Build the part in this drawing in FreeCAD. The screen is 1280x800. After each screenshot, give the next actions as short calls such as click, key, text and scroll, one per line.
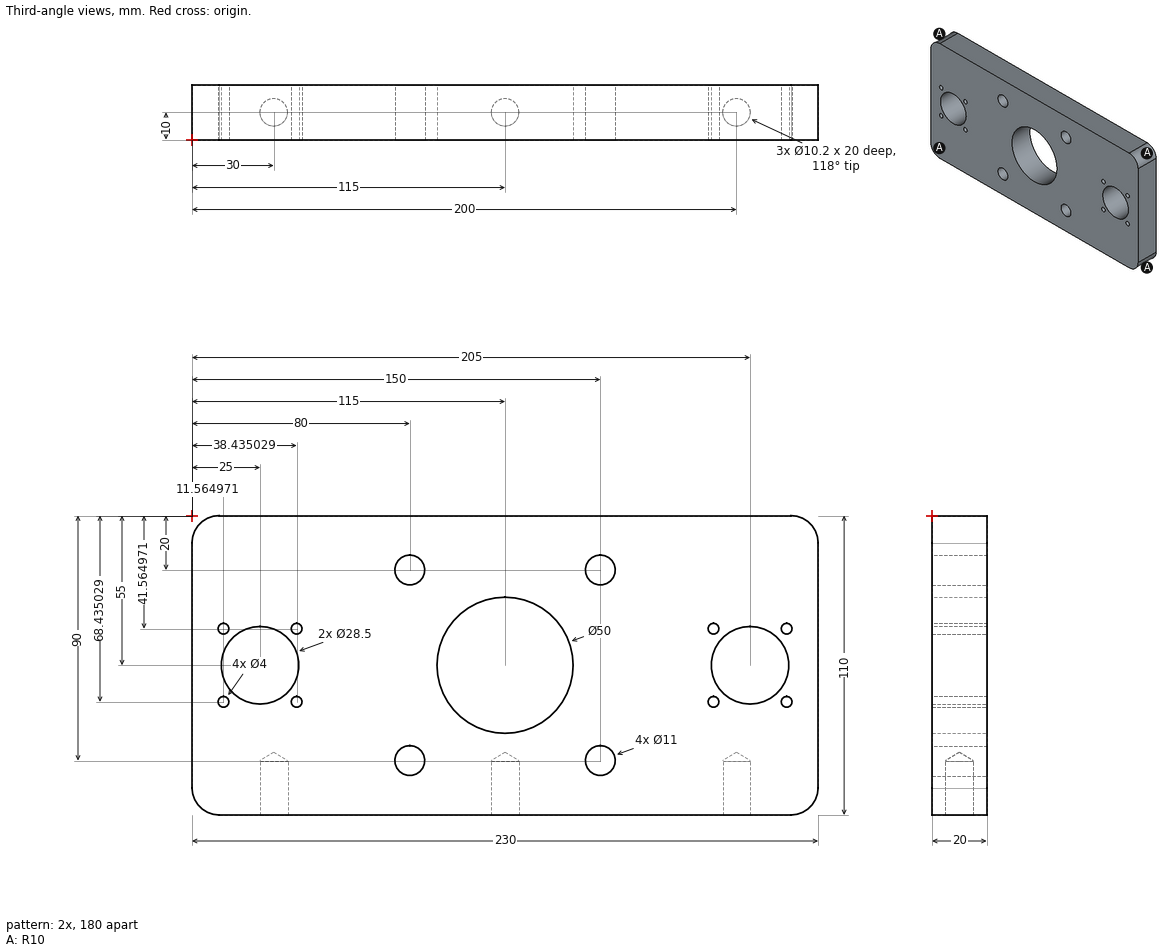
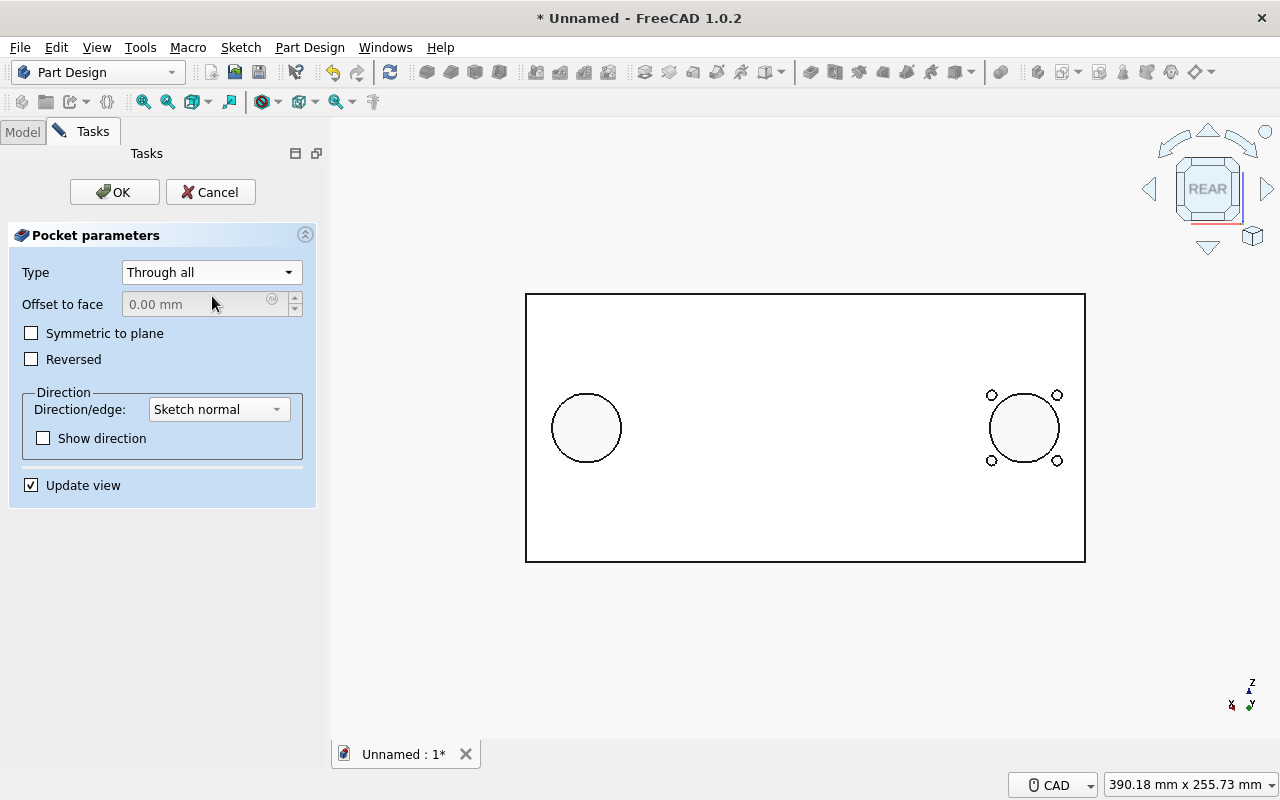
click(115, 192)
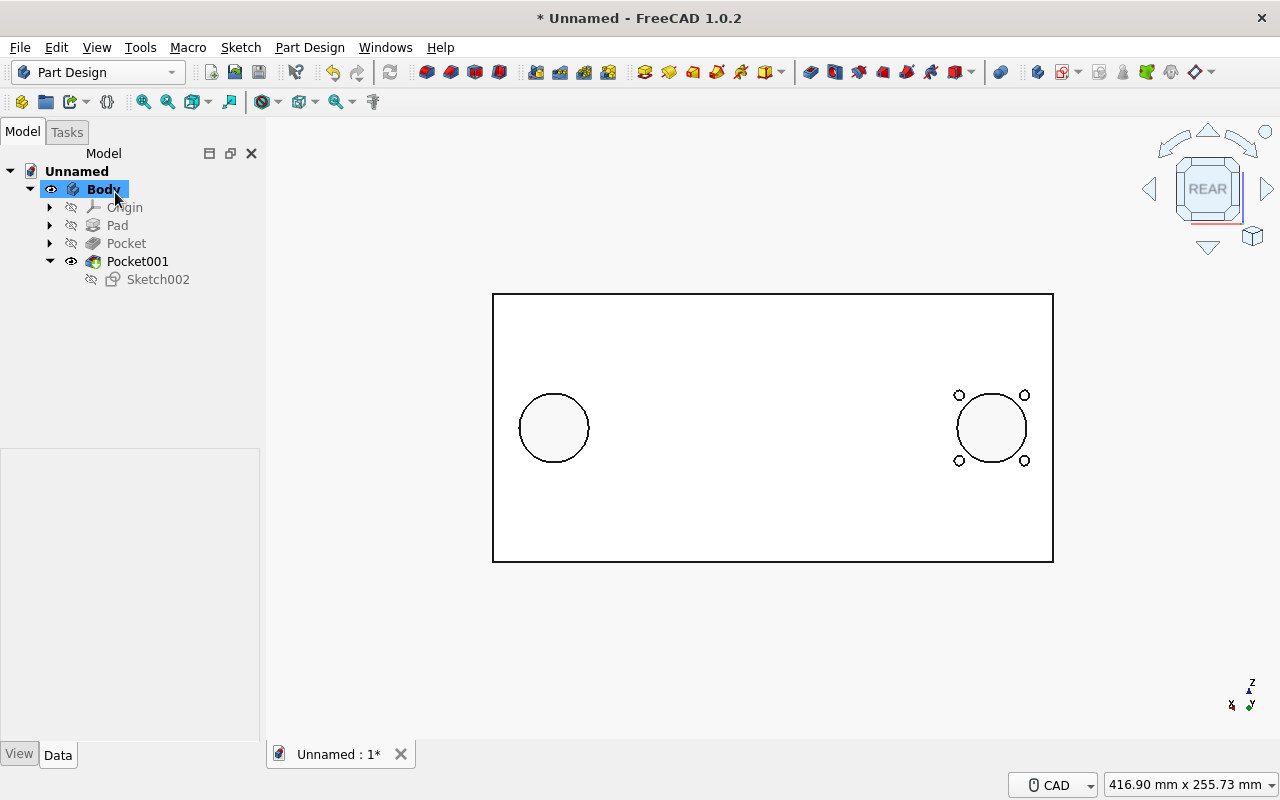
click(116, 261)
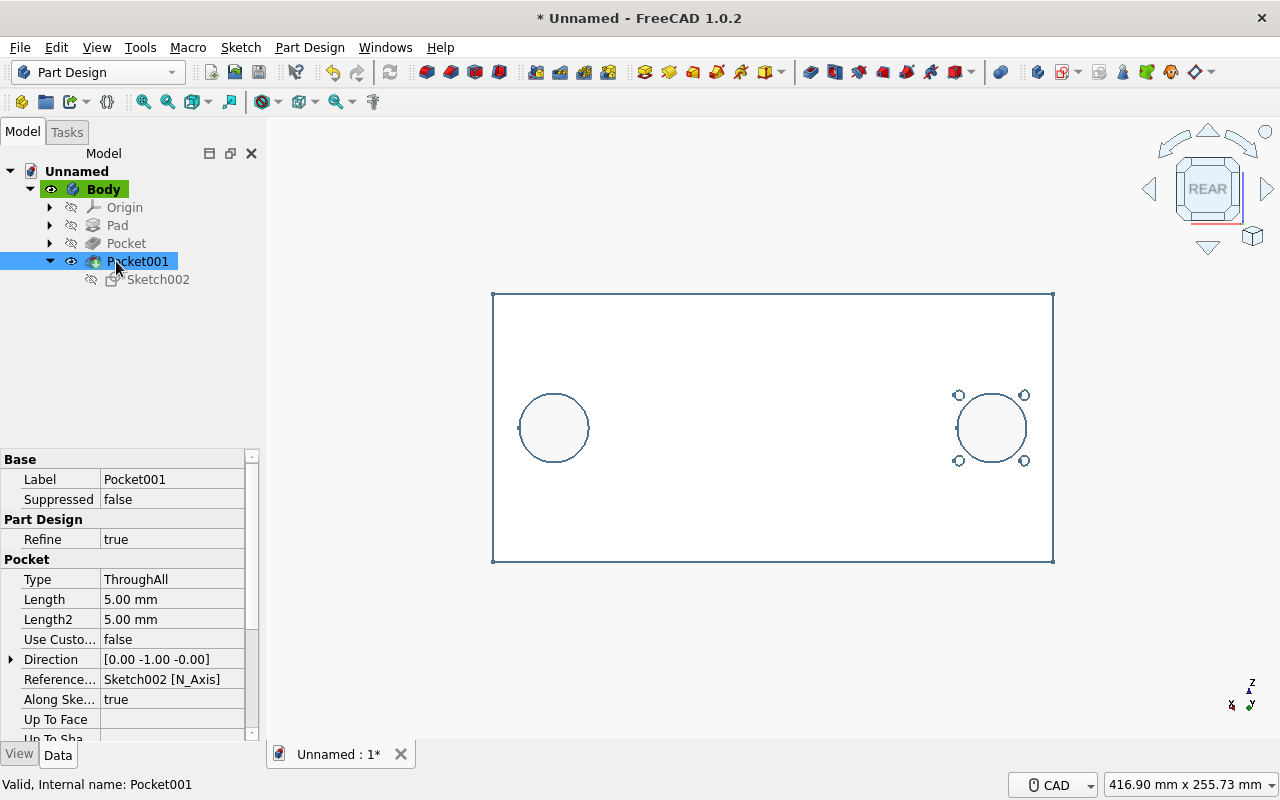
click(560, 72)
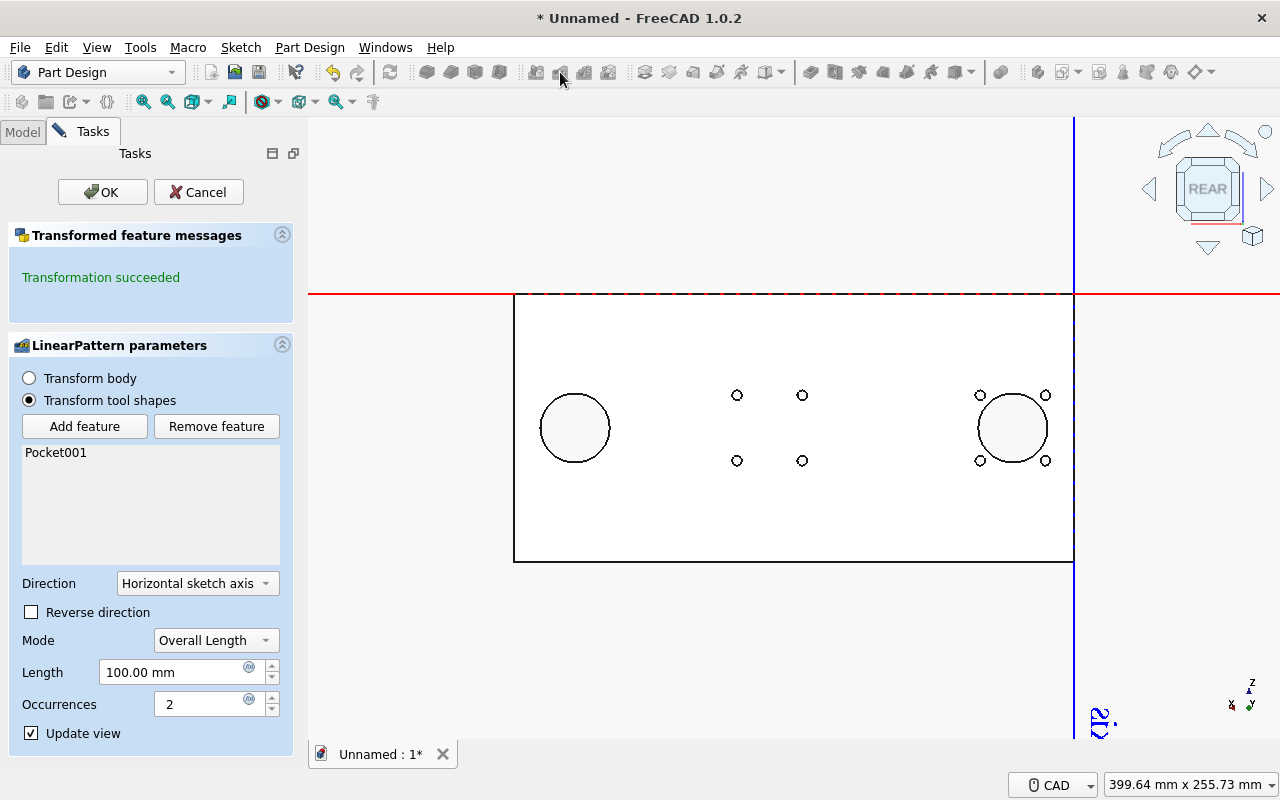
click(198, 584)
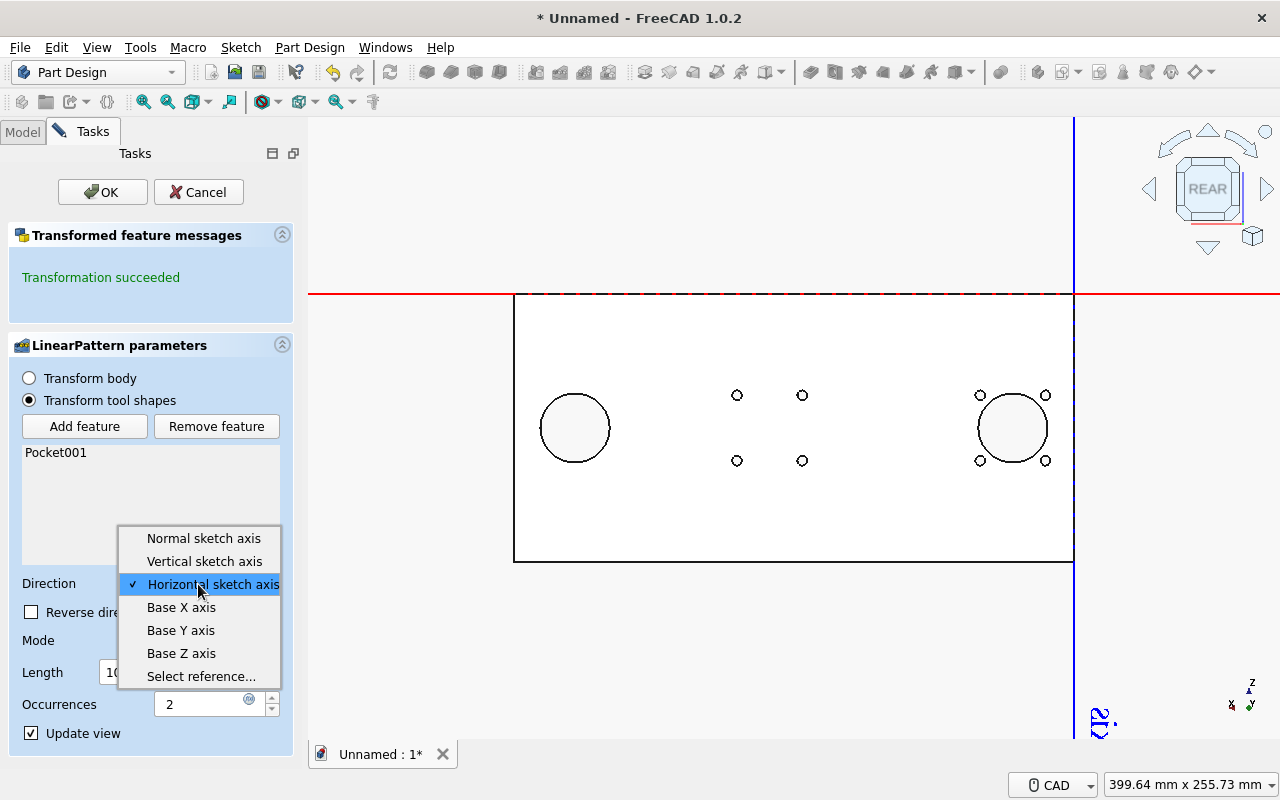
click(198, 608)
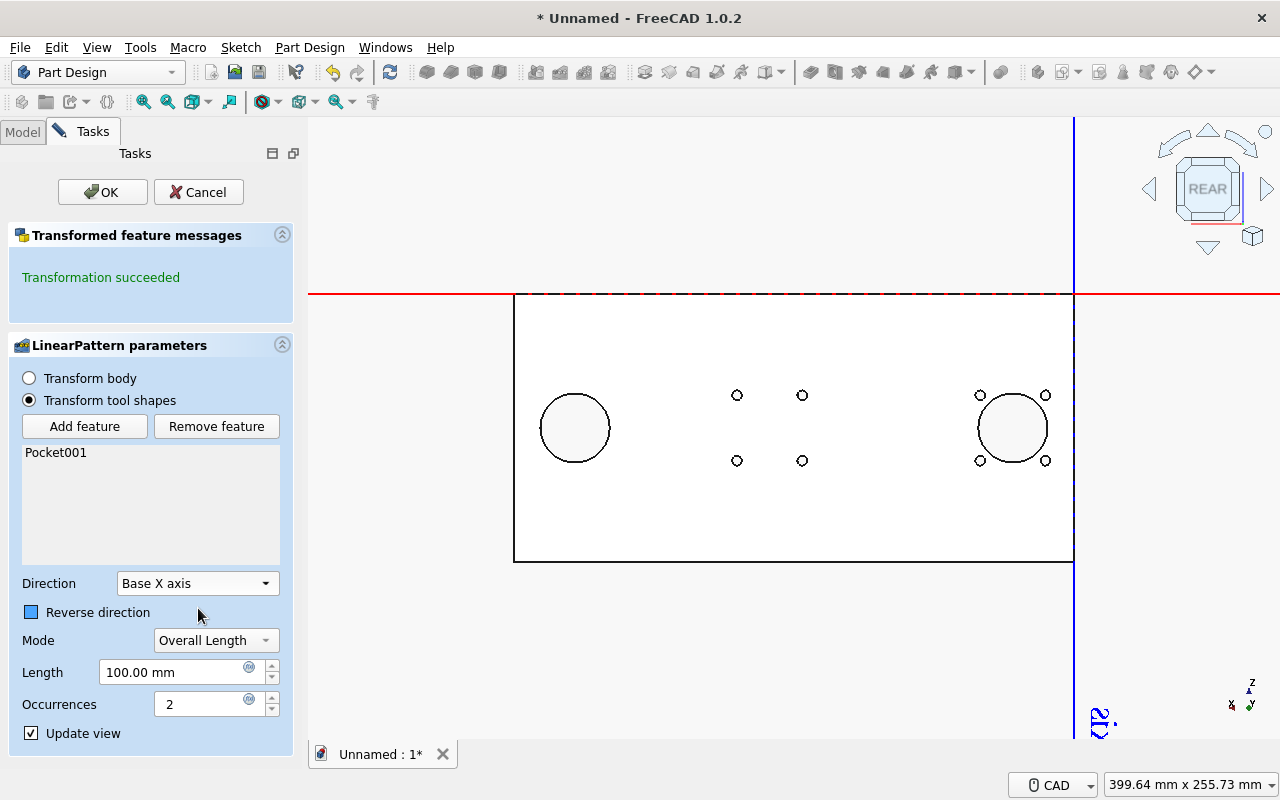
click(217, 640)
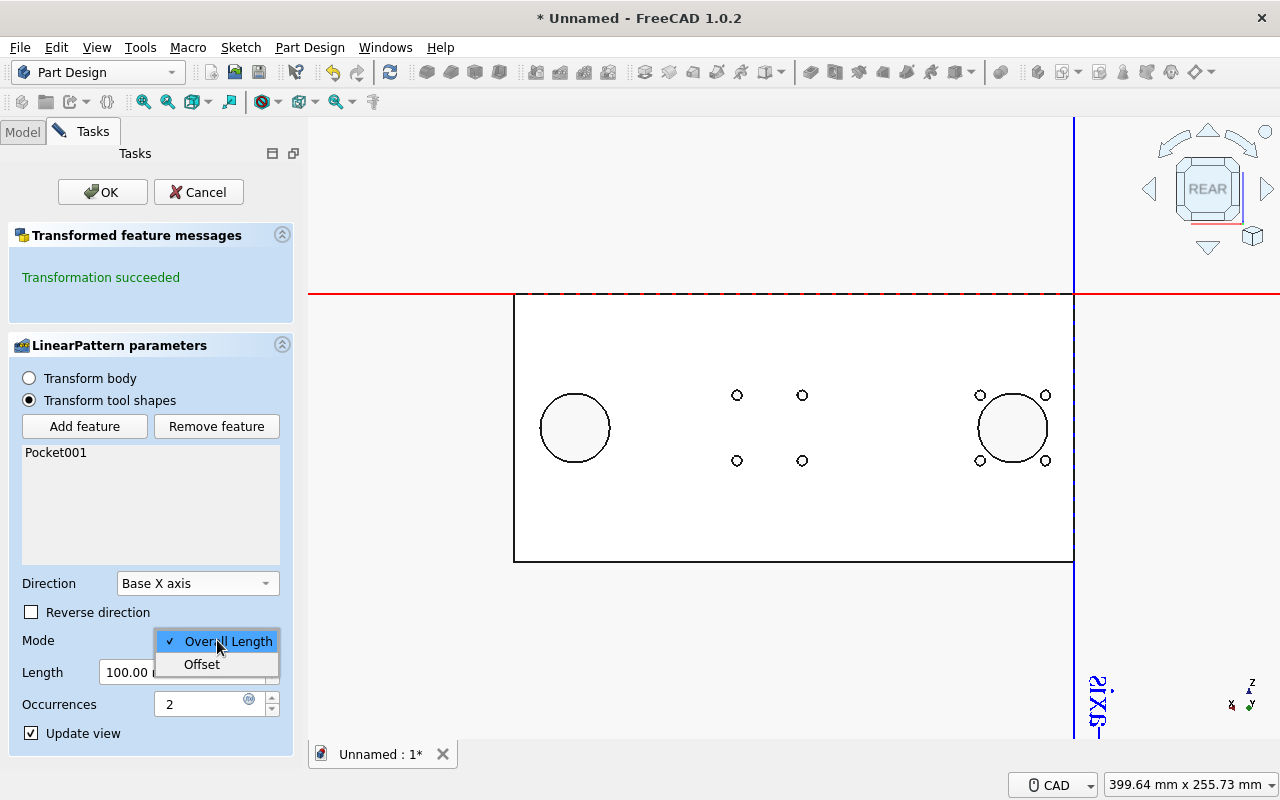
click(216, 664)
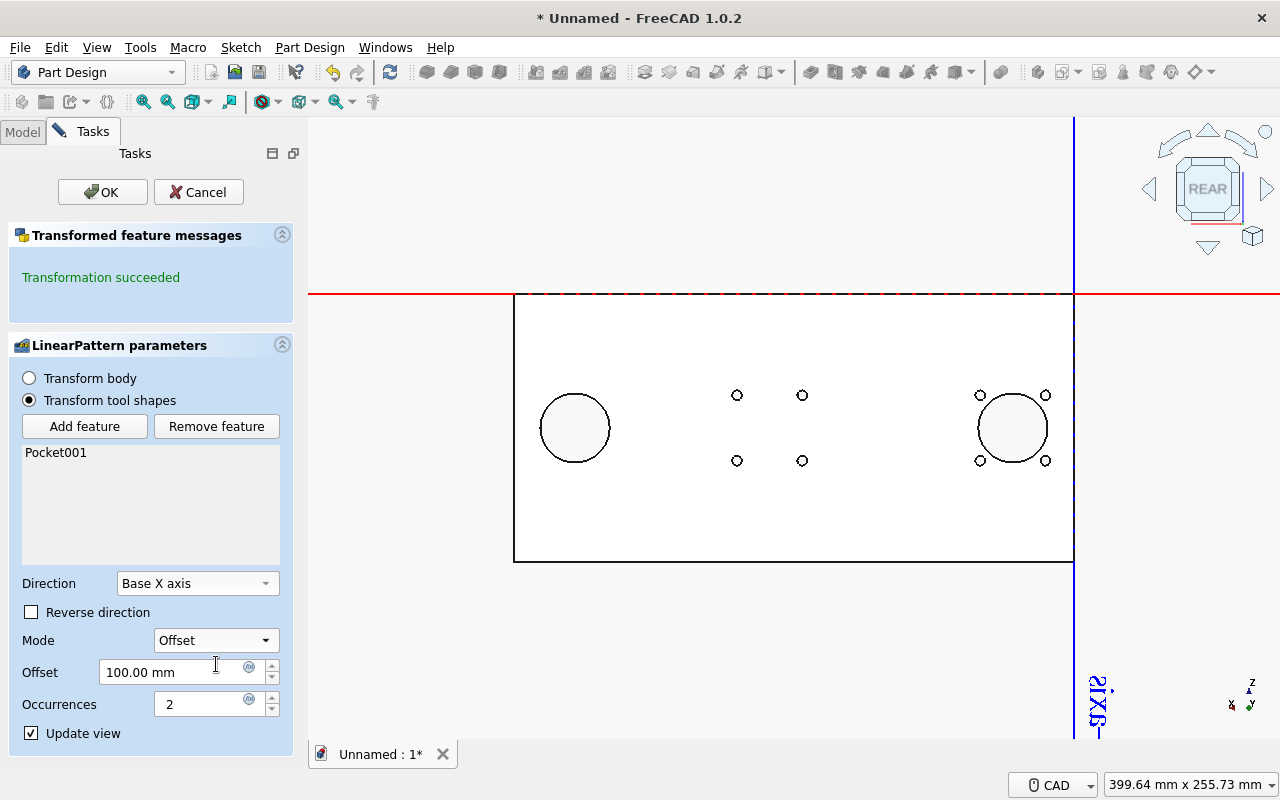
triple_click(182, 672)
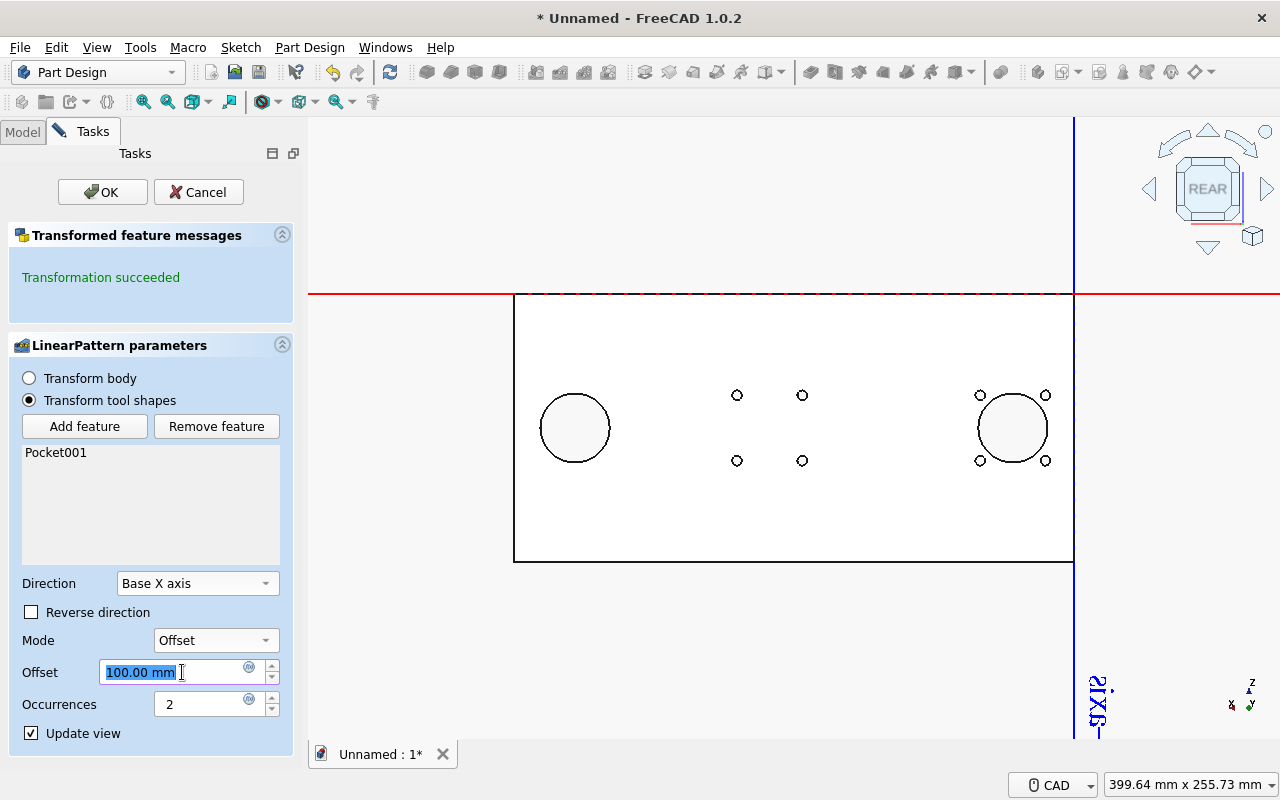
text(180)
key(Tab)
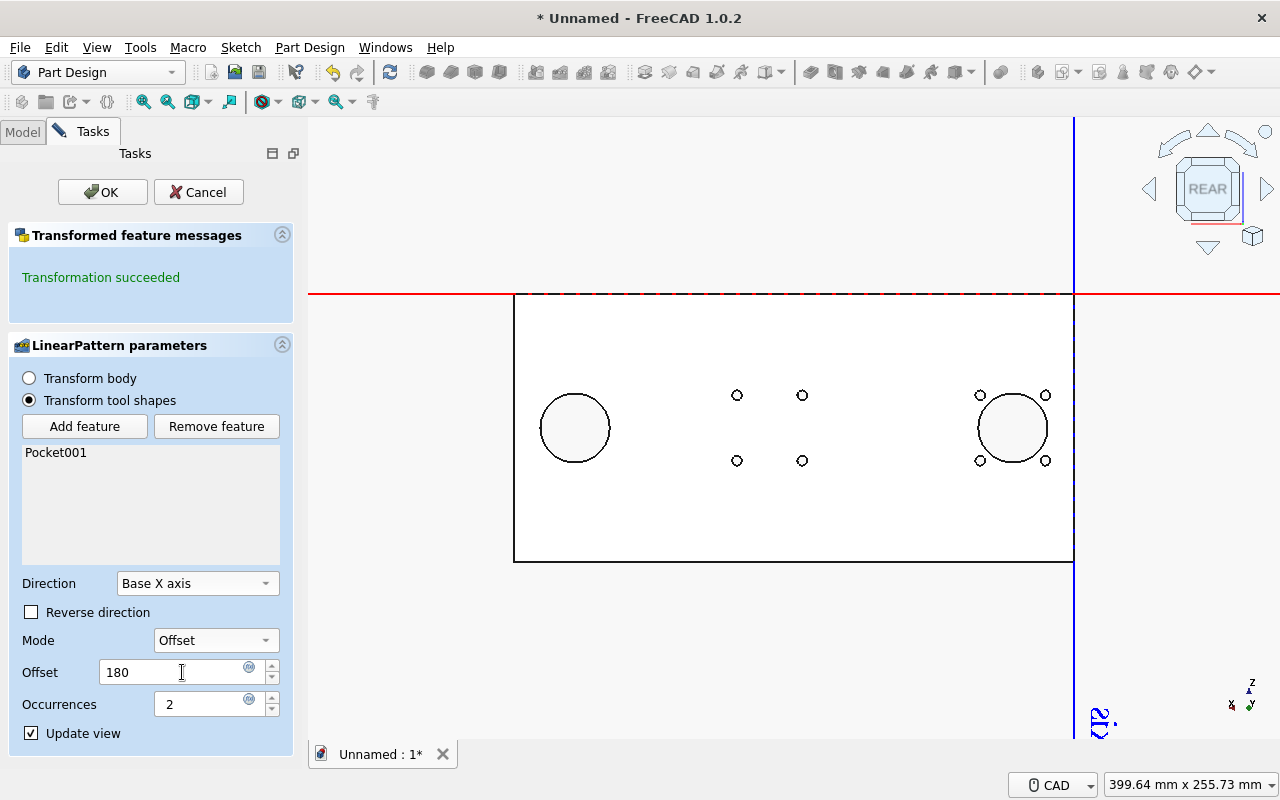
triple_click(209, 704)